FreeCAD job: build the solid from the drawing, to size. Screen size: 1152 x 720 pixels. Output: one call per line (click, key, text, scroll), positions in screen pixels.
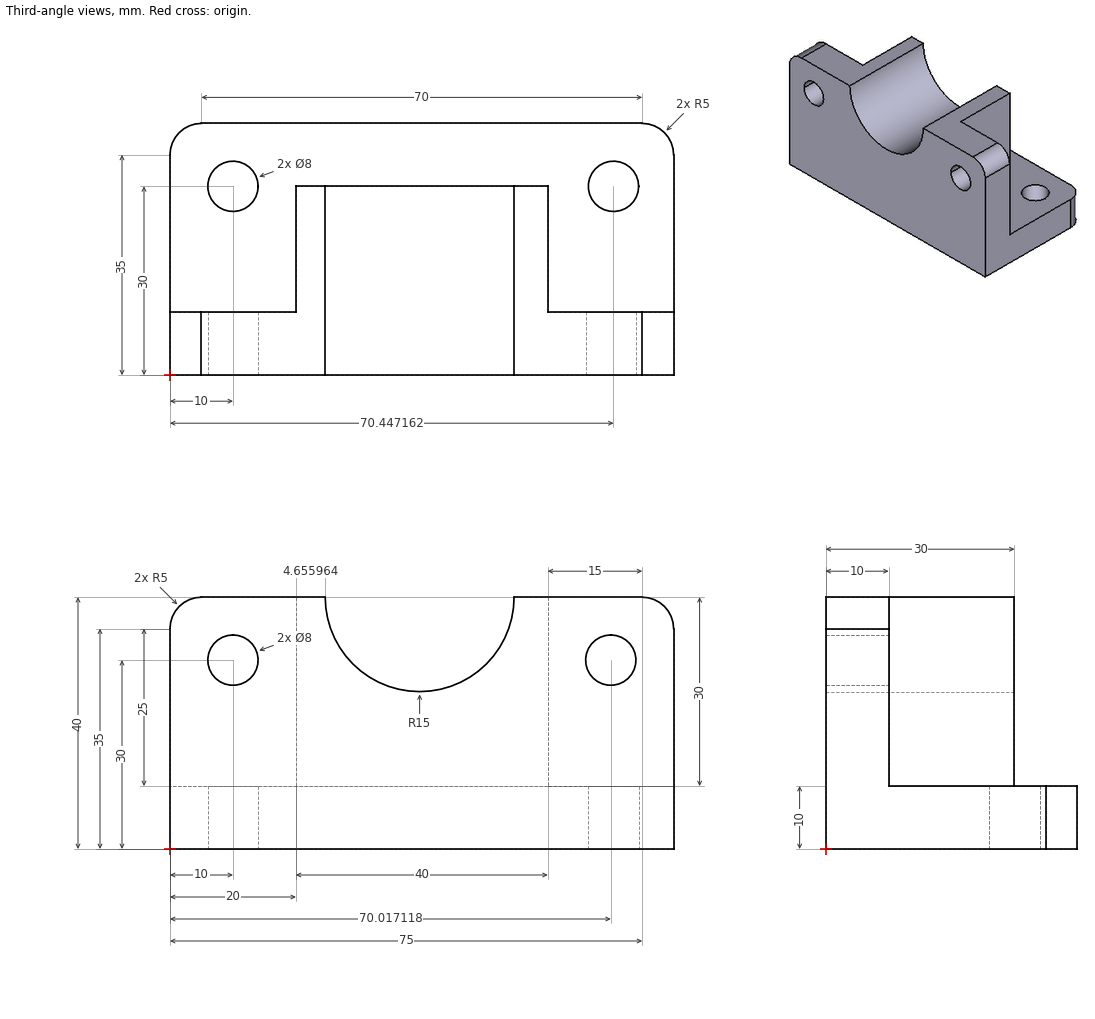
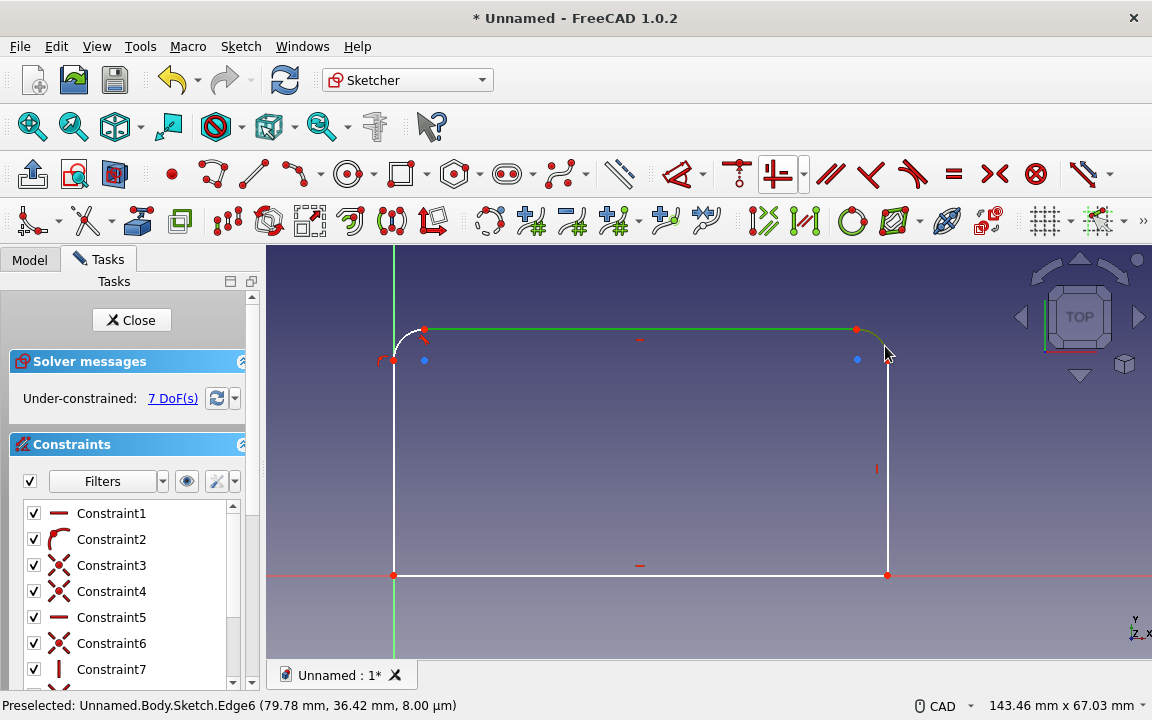
click(913, 174)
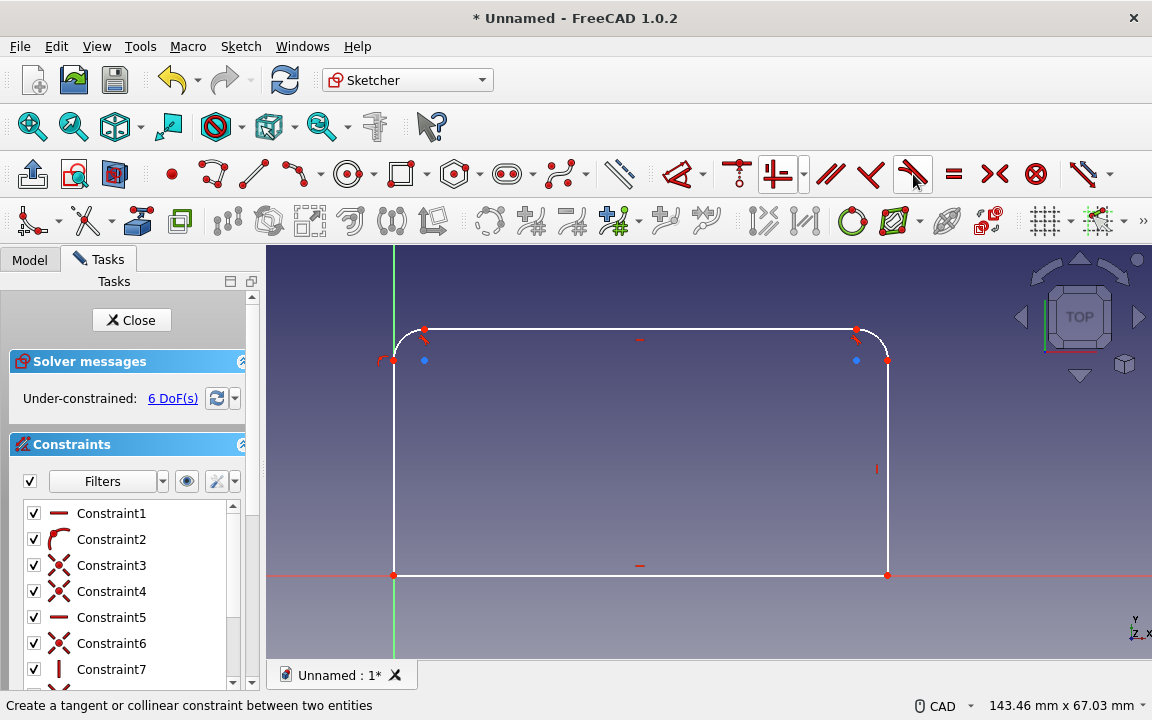
click(394, 425)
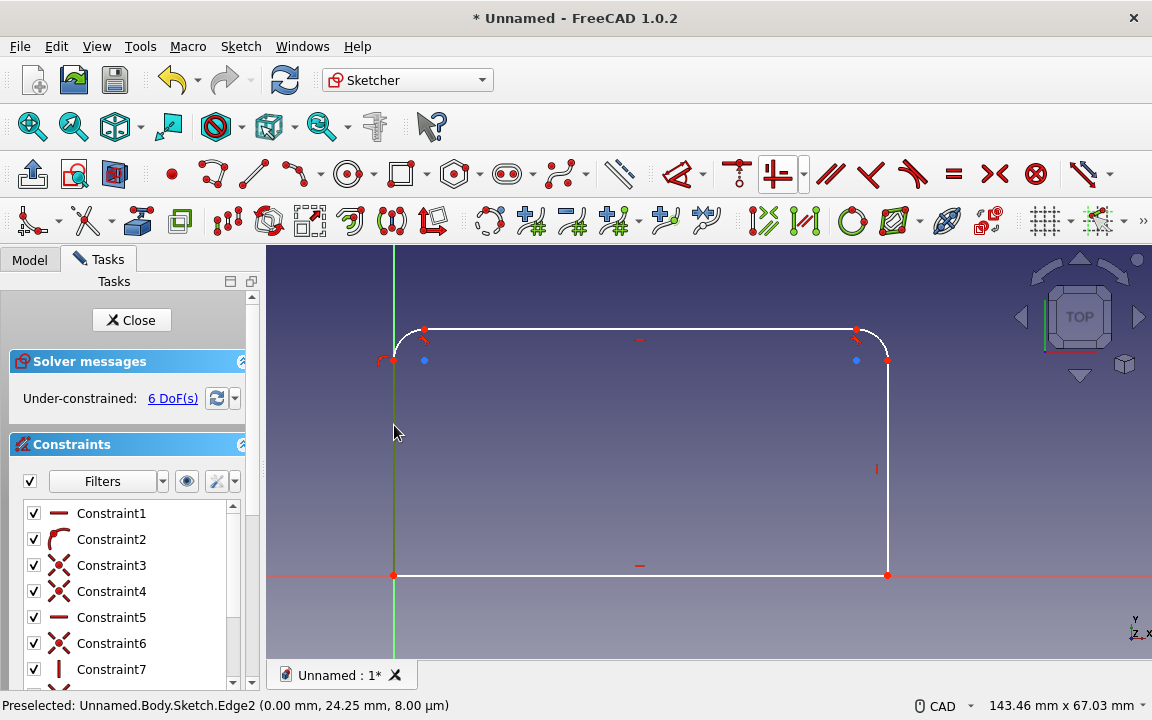
click(411, 333)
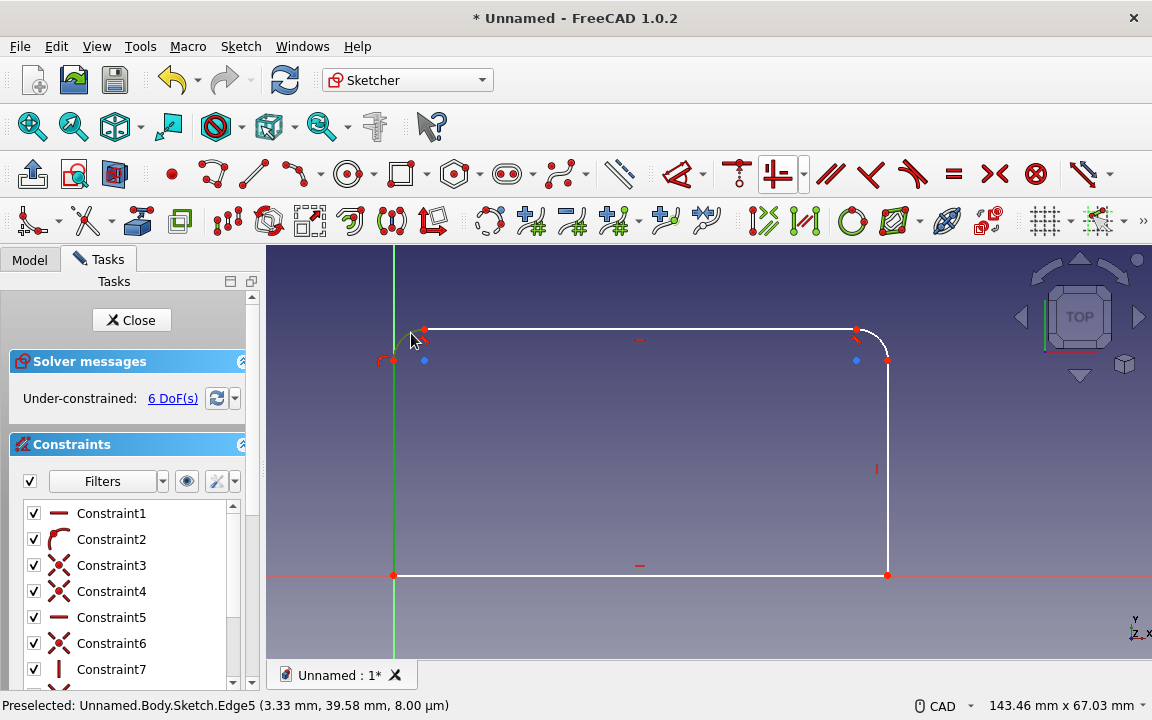
click(913, 174)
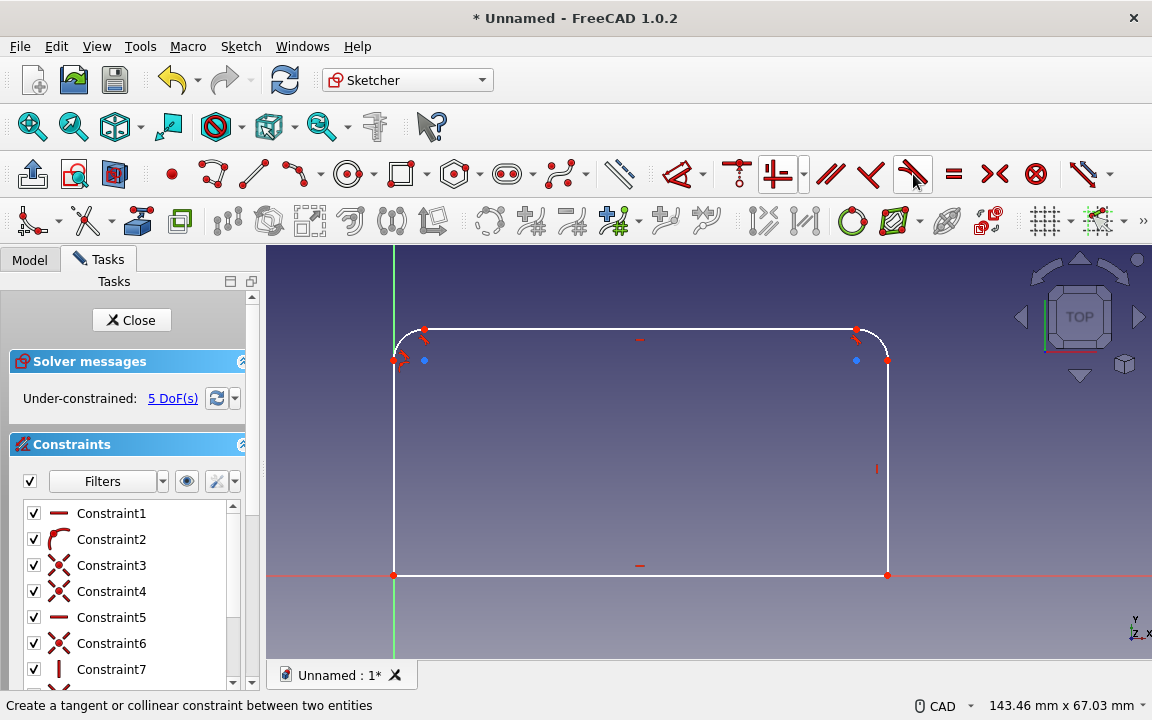
click(888, 511)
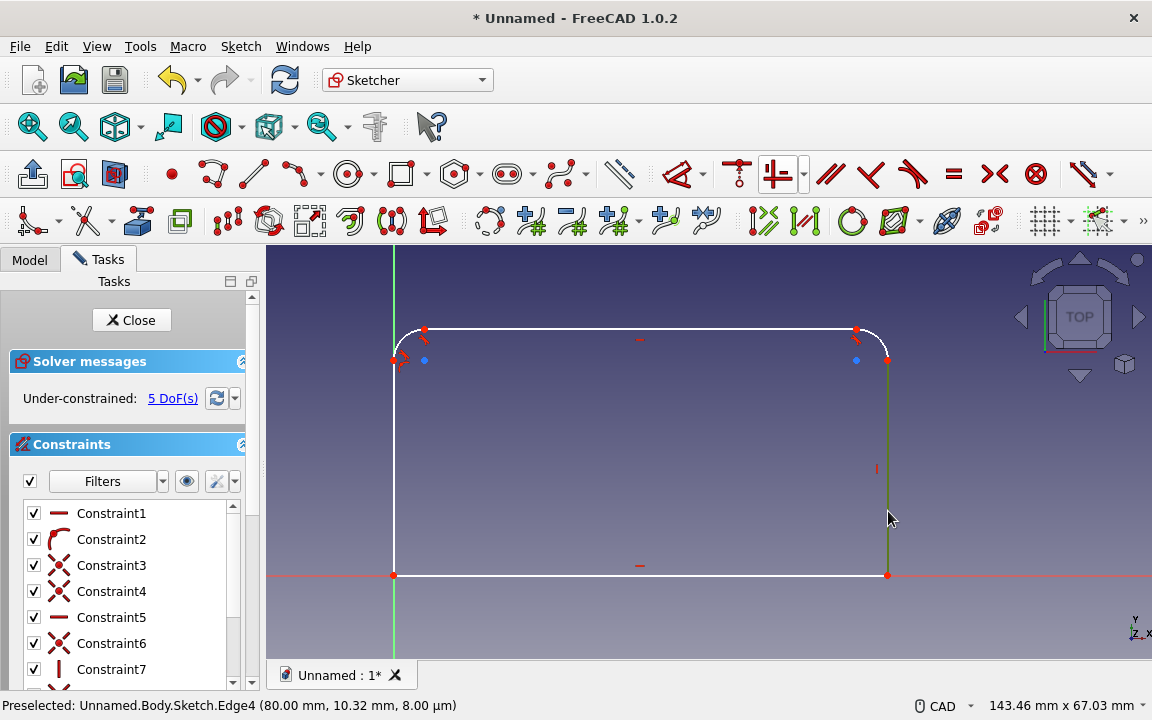
click(885, 346)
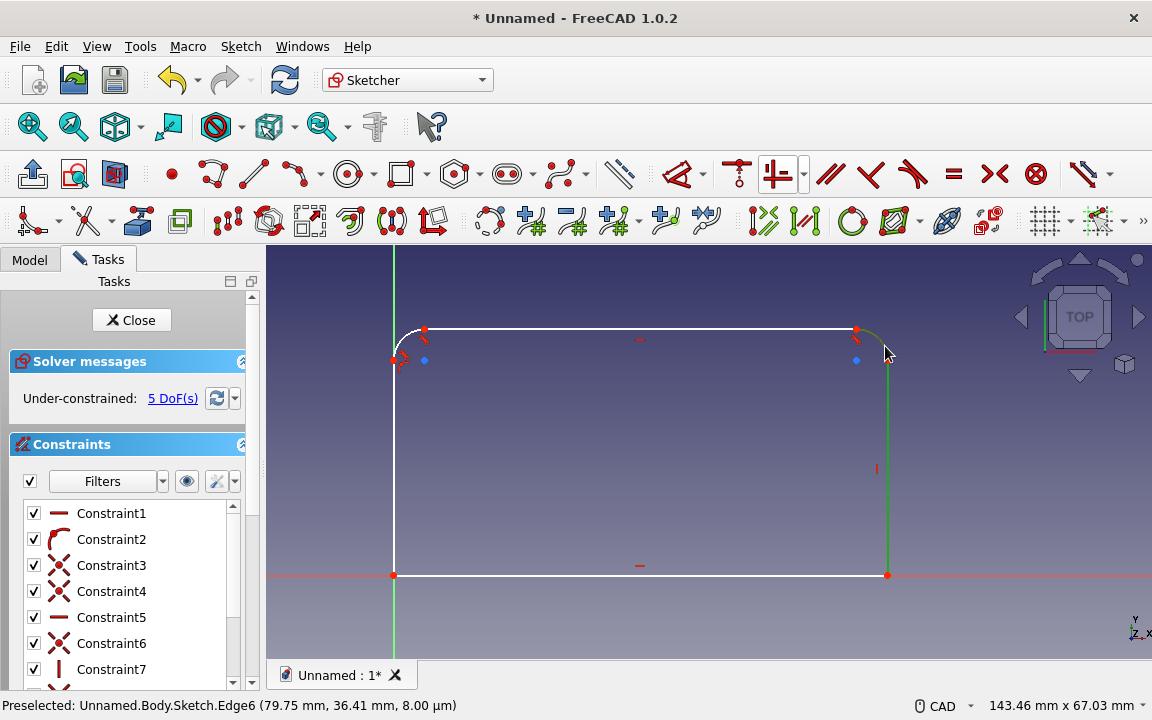
key(t)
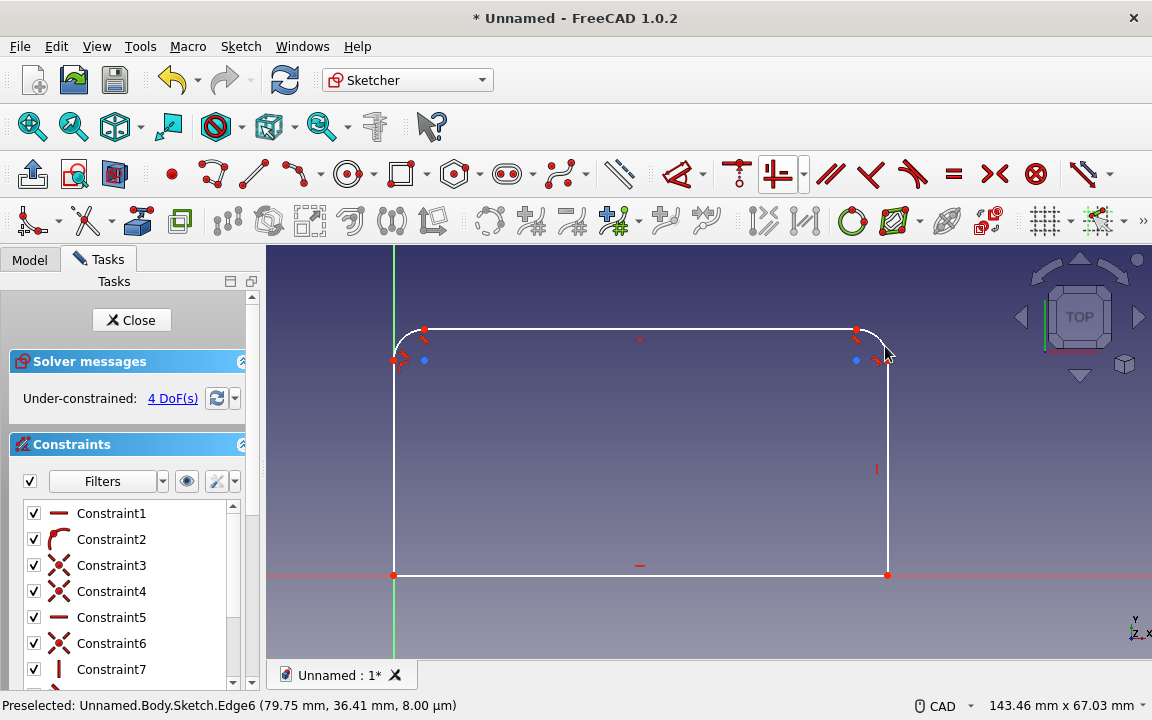
click(411, 333)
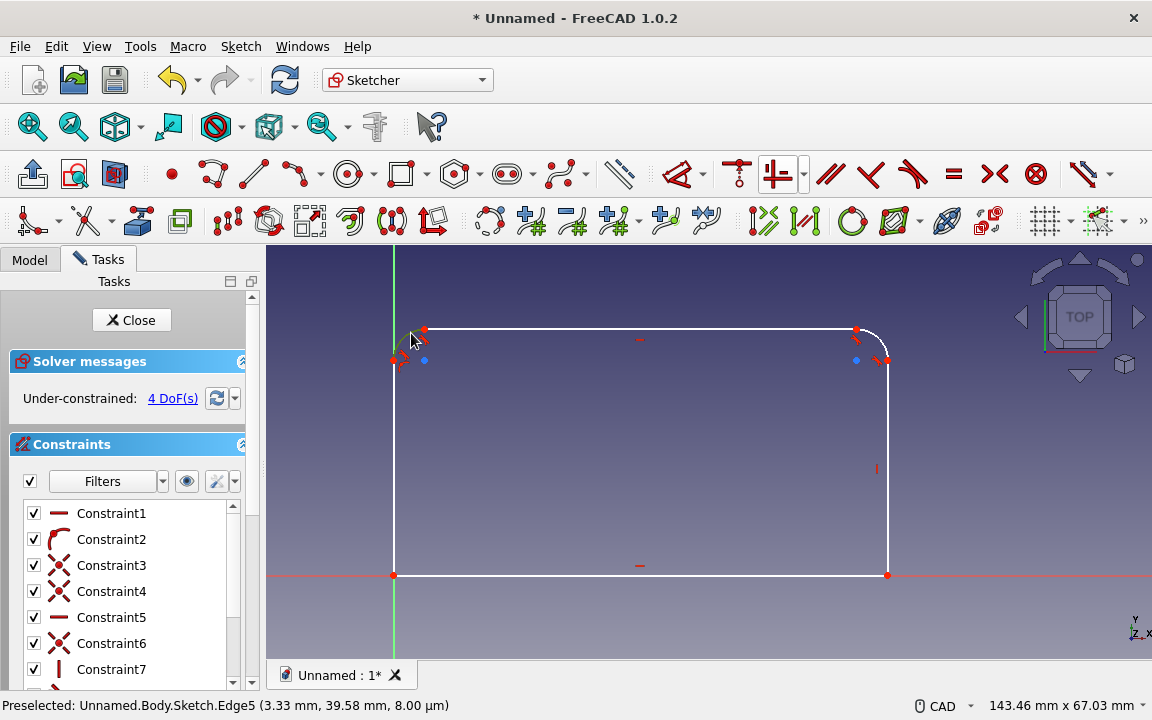
click(885, 346)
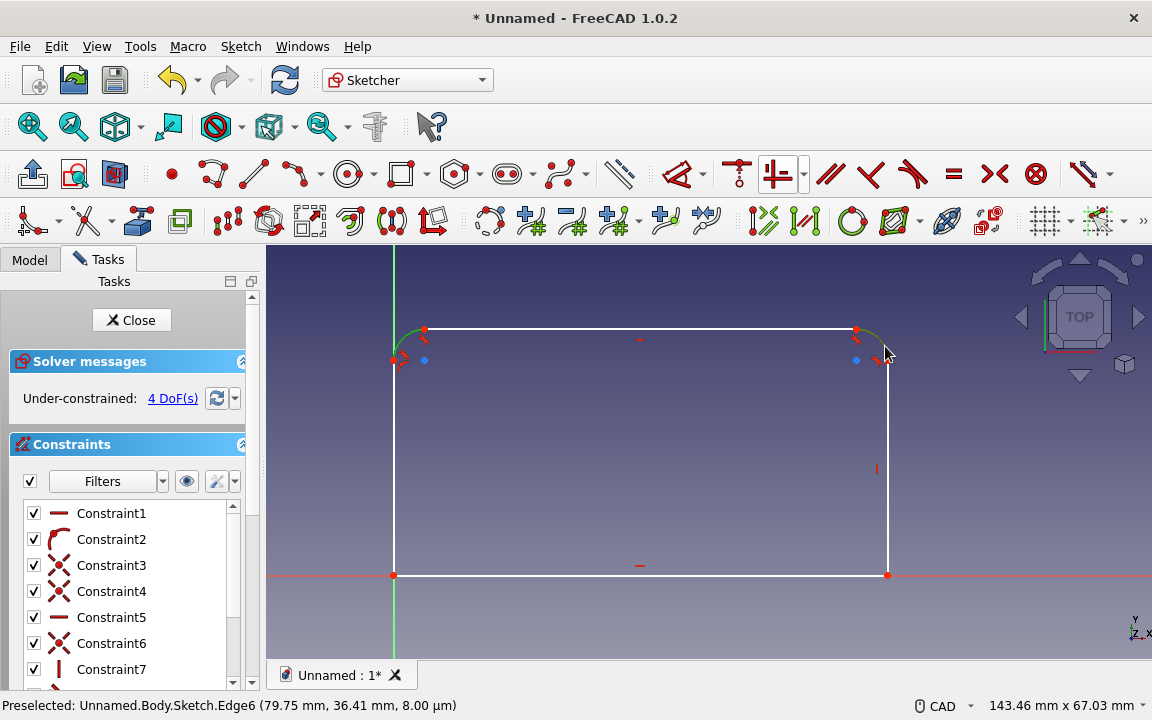
key(e)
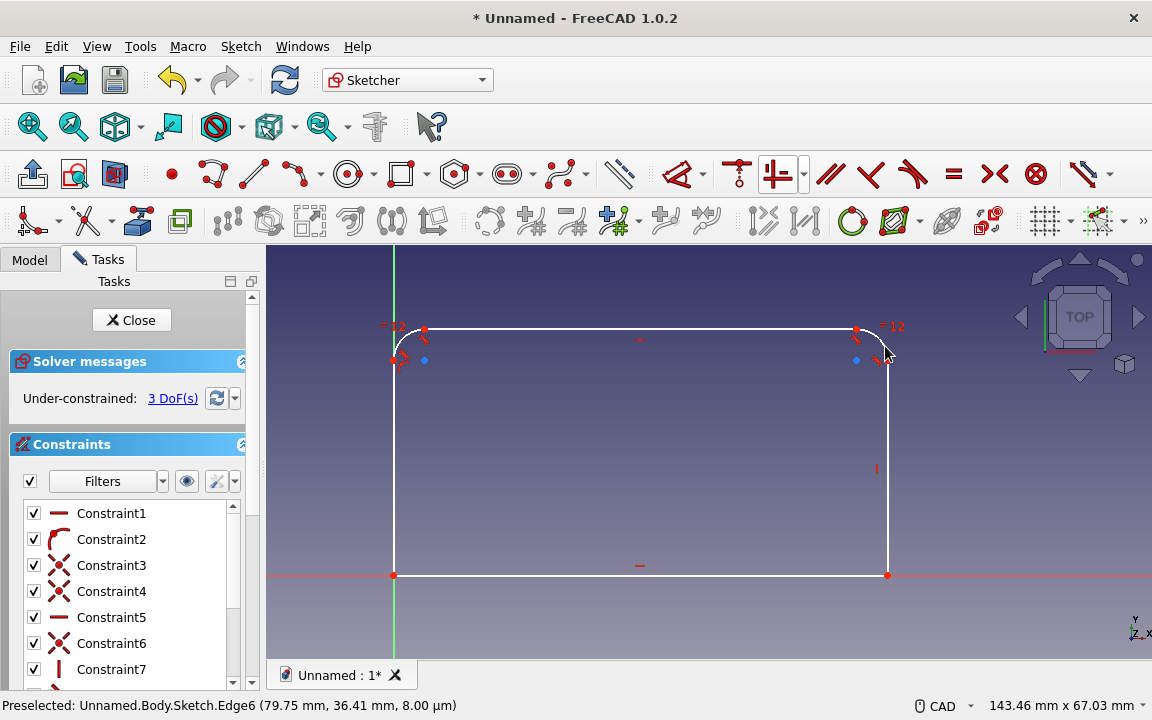
click(676, 174)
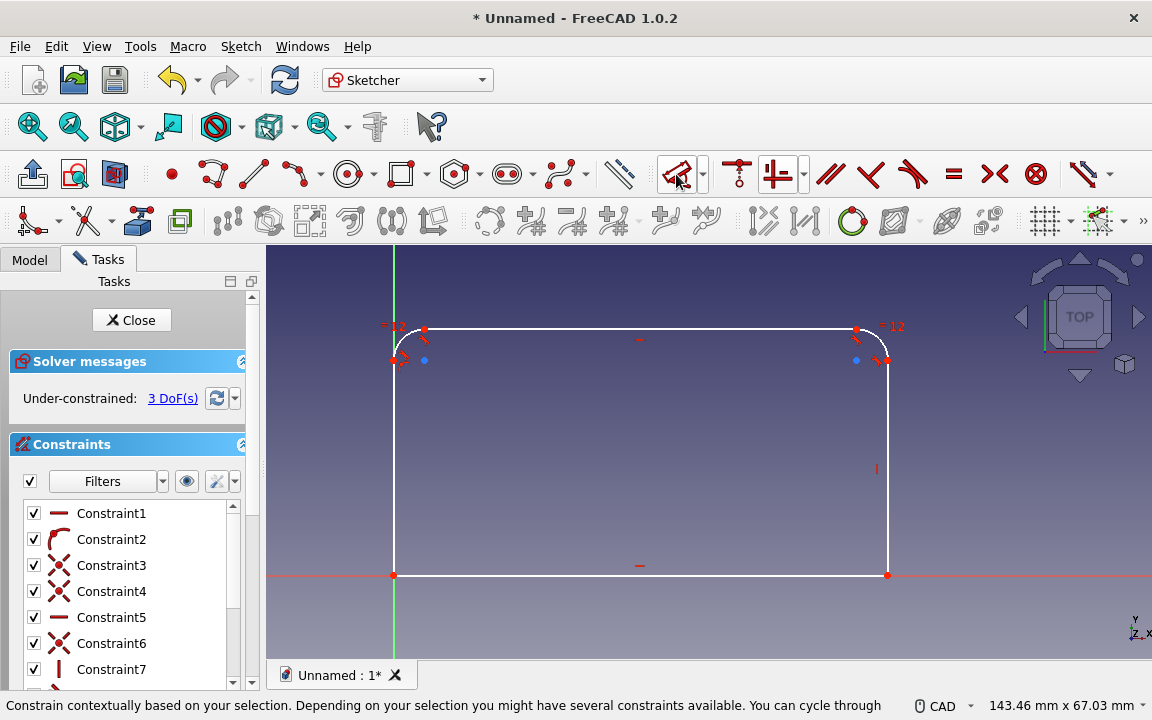
scroll(411, 333, up, 2)